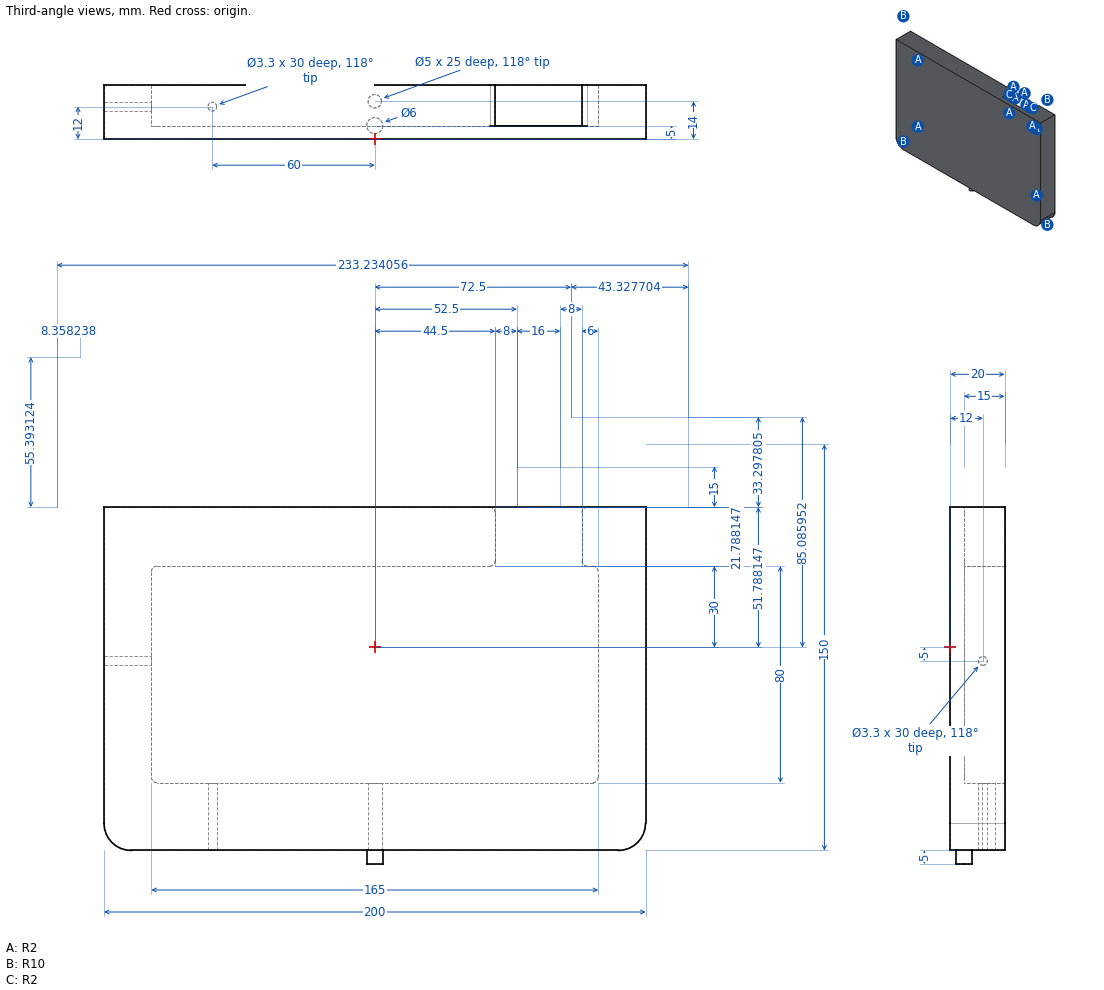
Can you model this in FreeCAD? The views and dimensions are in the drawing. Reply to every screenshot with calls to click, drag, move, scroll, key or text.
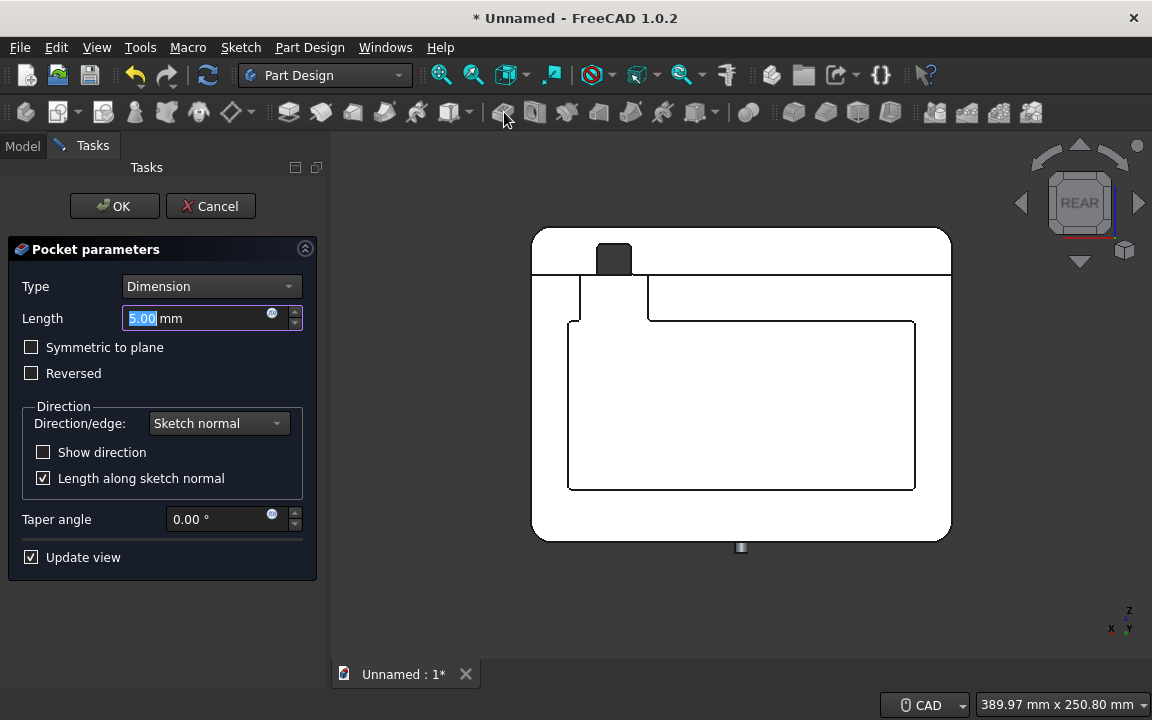
click(212, 286)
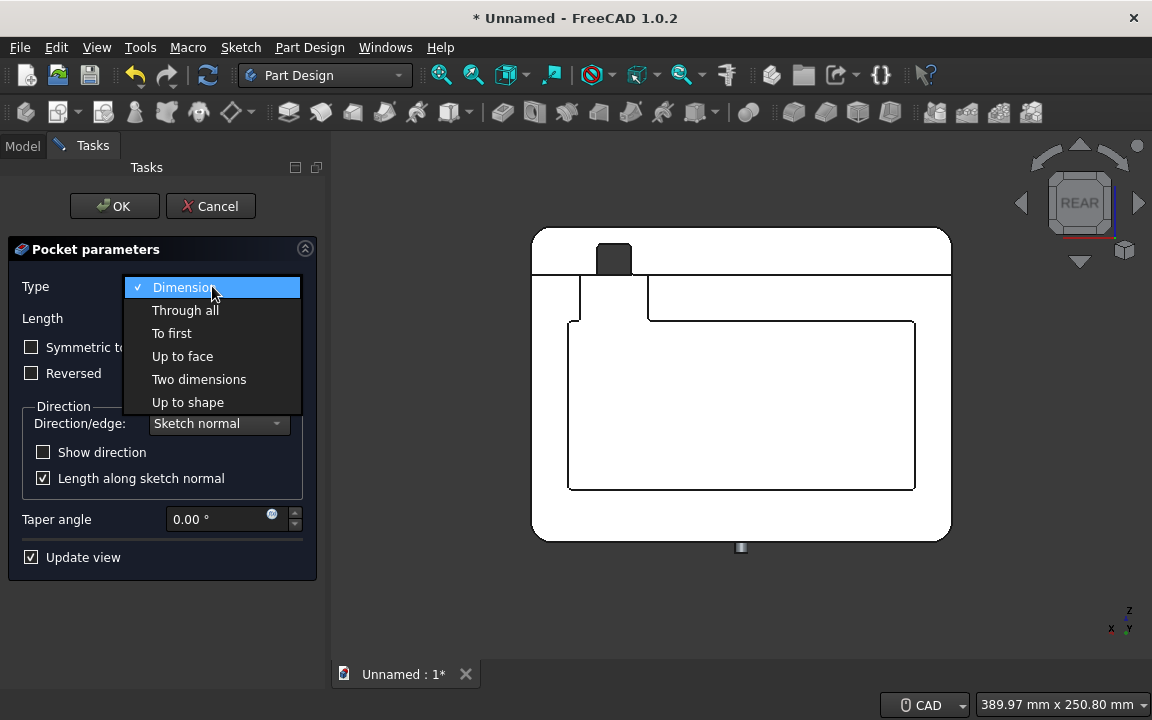
click(212, 310)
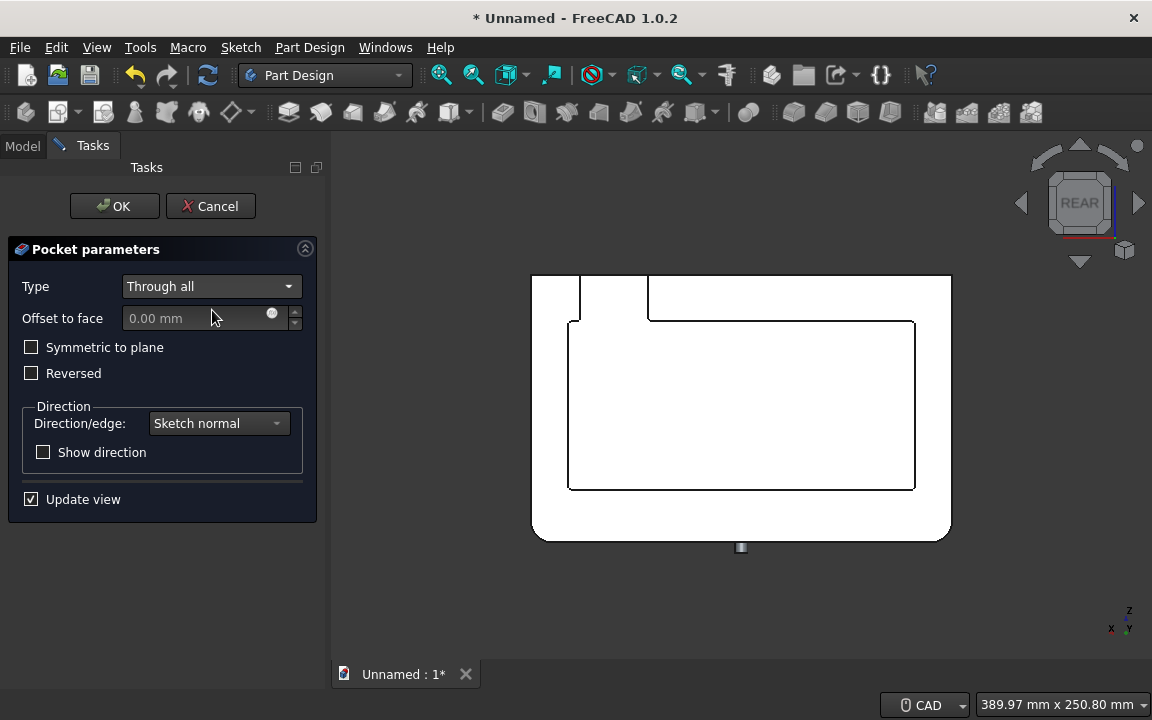
click(115, 206)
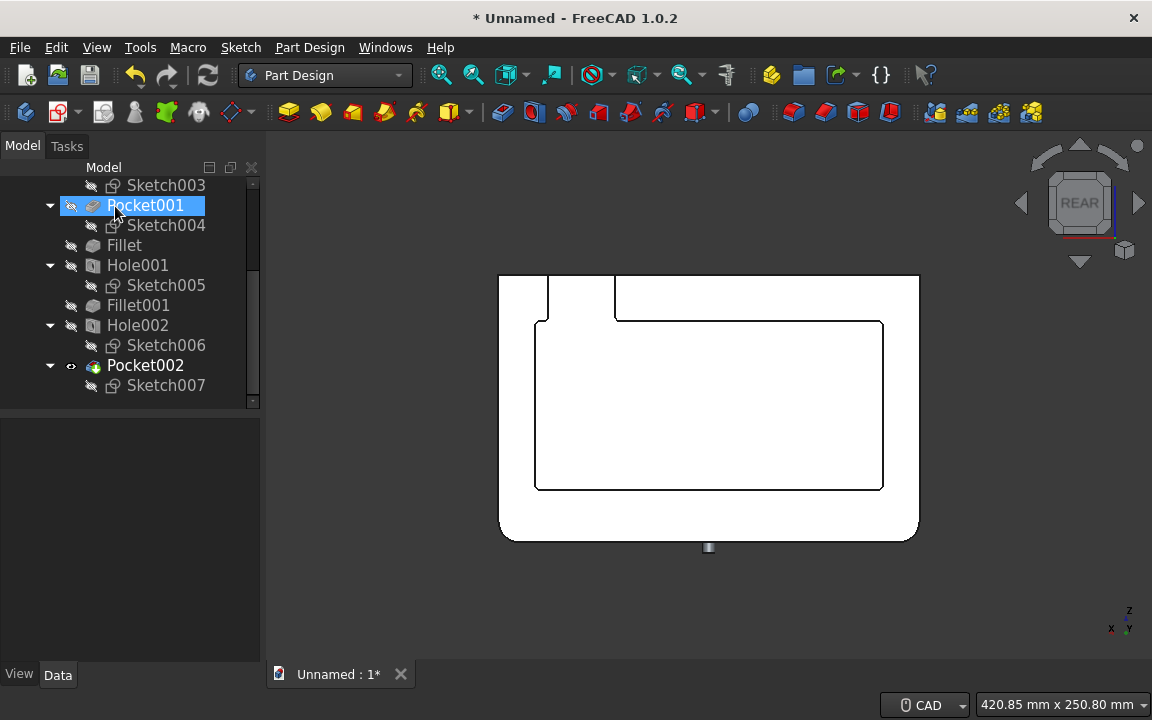
key(0)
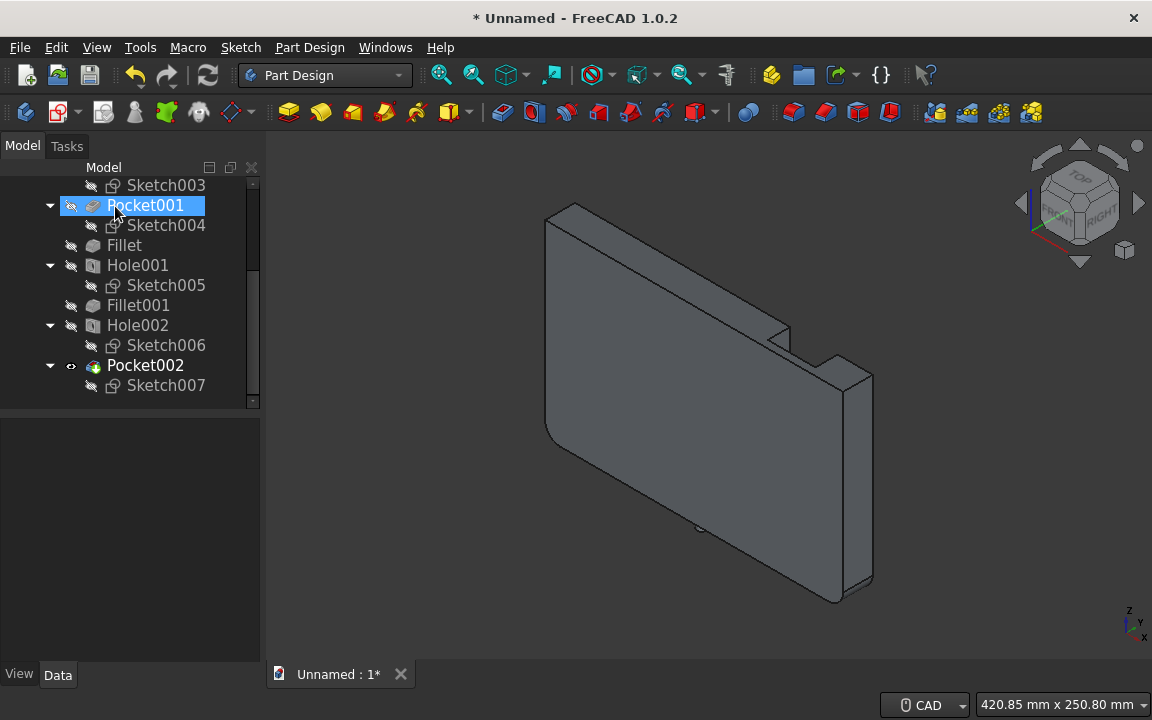
click(779, 332)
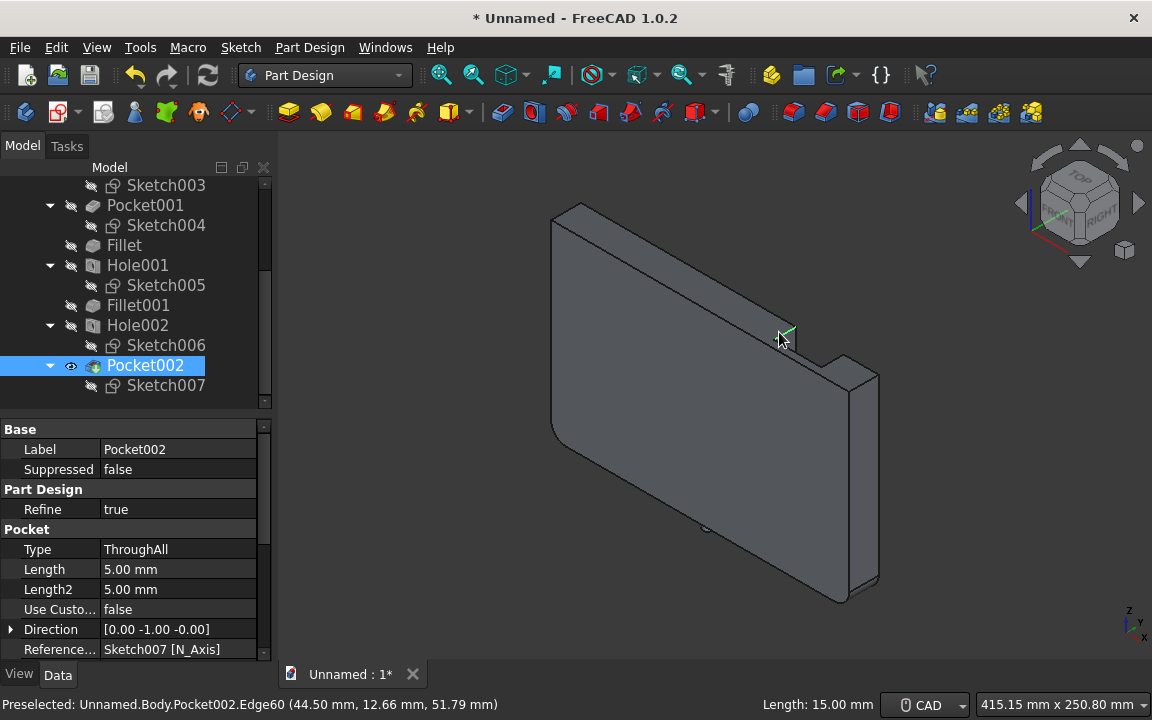
key(2)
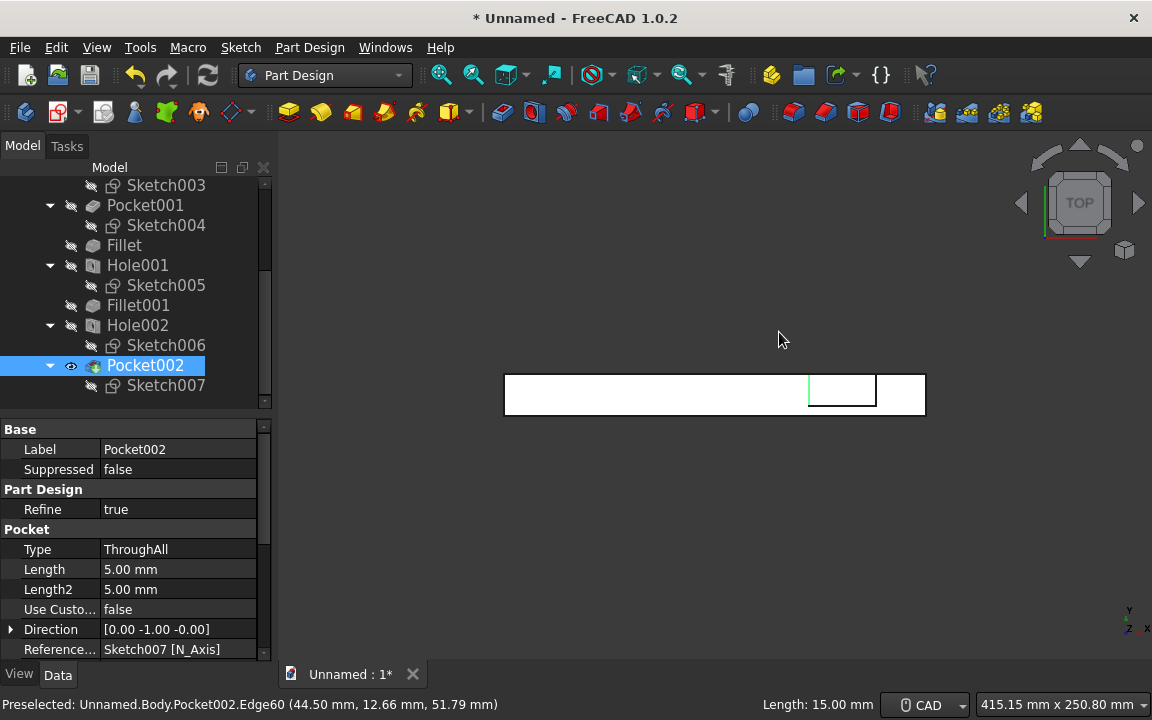
click(876, 389, ctrl)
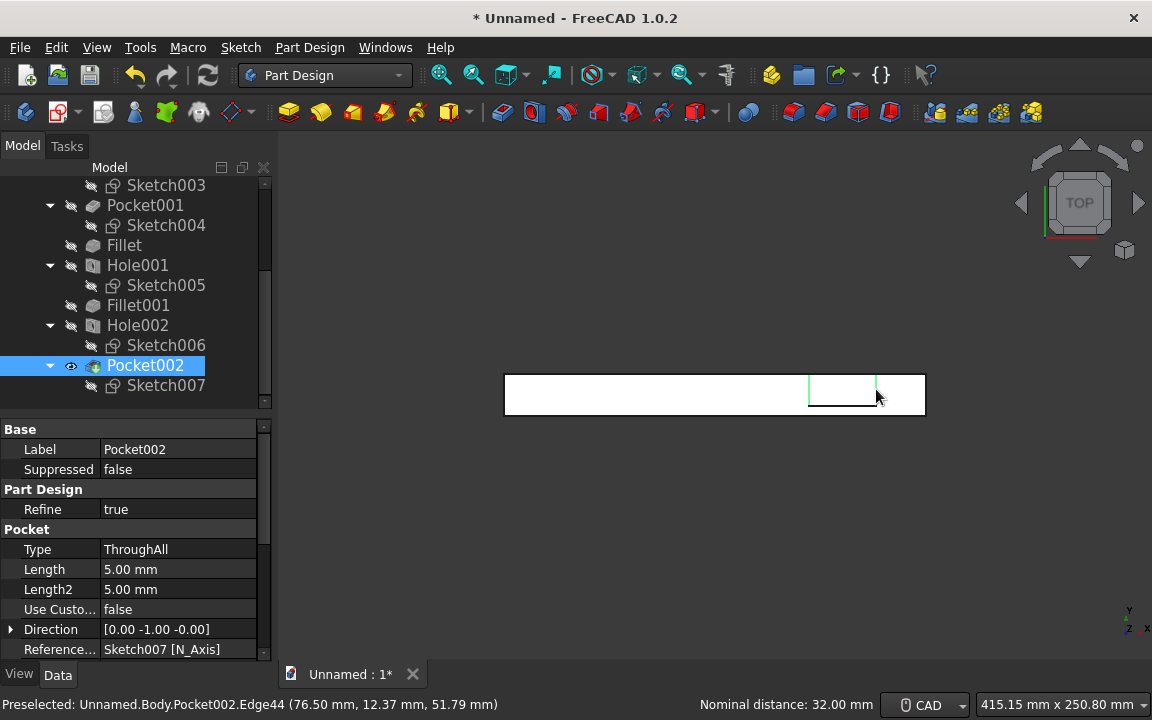
click(794, 112)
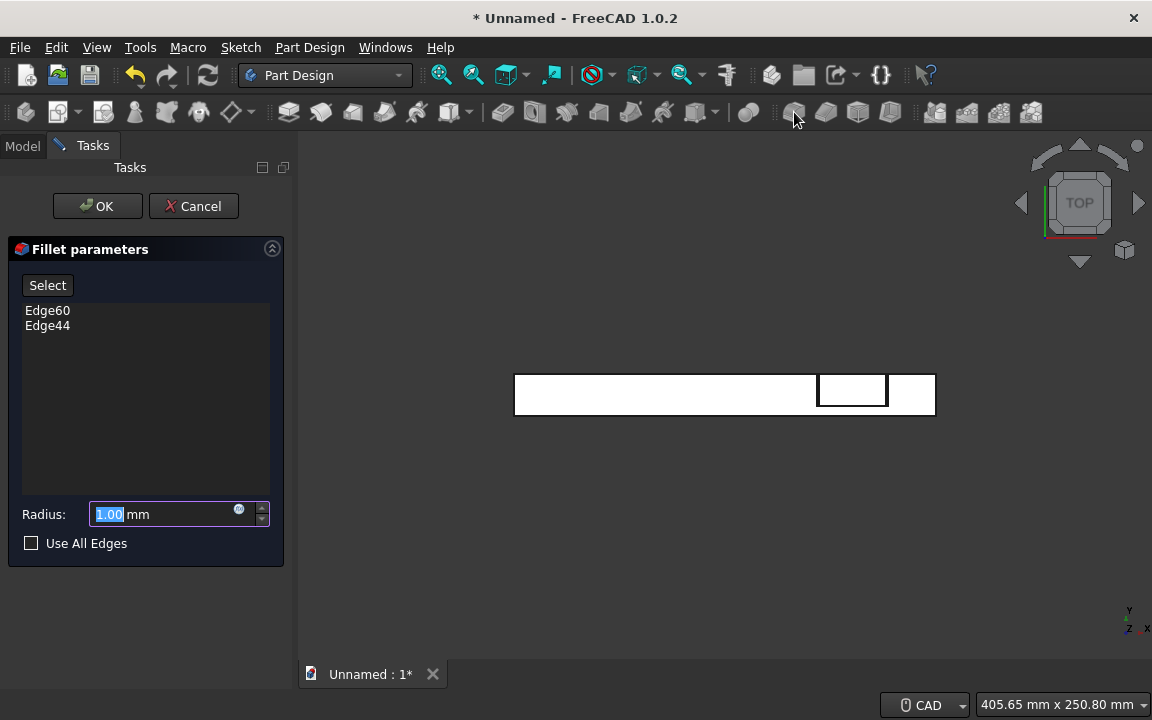
text(2)
key(Tab)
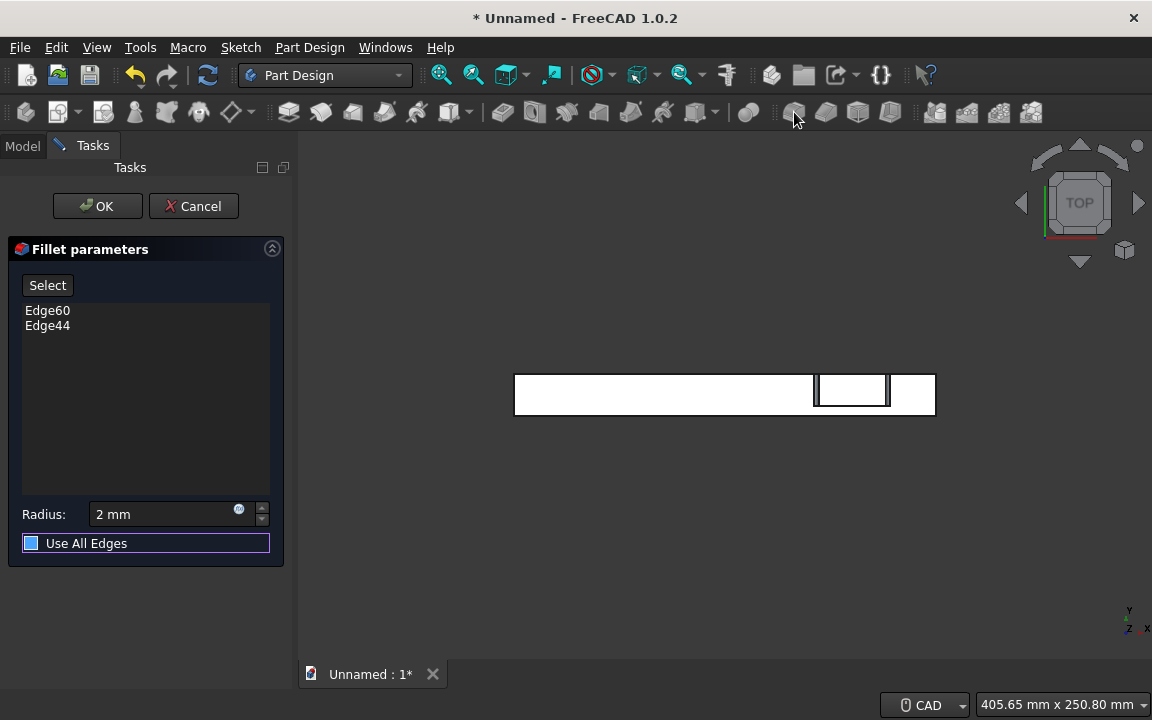
click(98, 206)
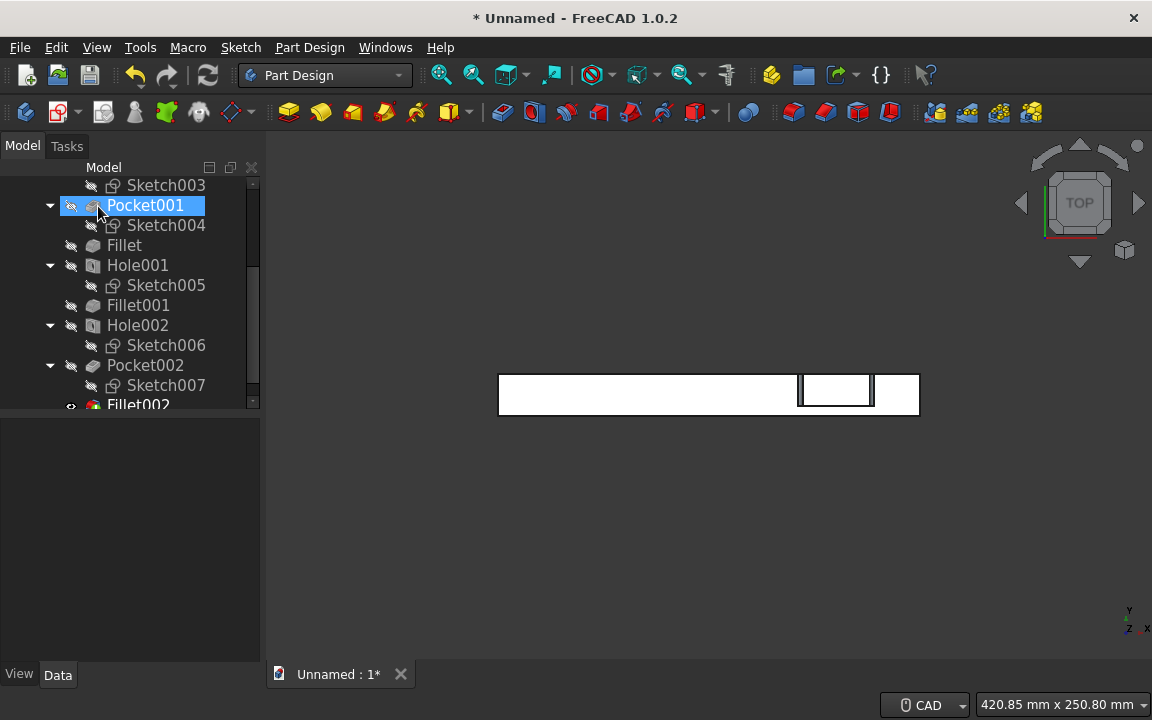
key(0)